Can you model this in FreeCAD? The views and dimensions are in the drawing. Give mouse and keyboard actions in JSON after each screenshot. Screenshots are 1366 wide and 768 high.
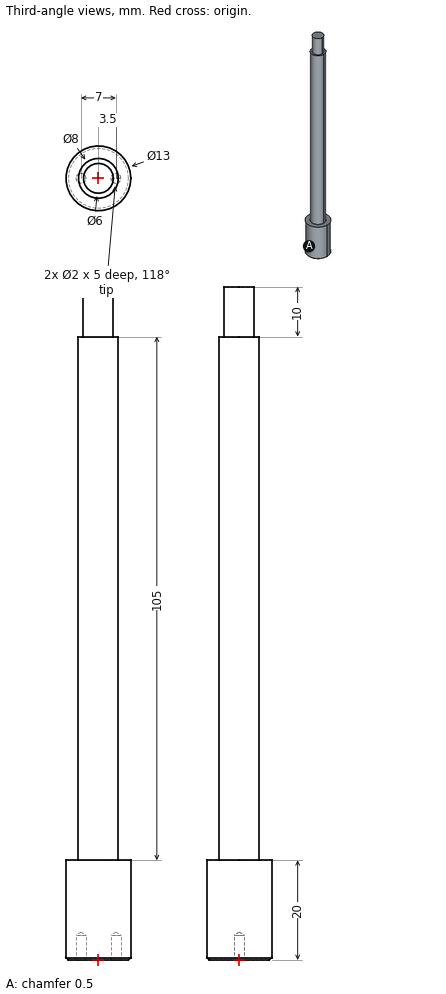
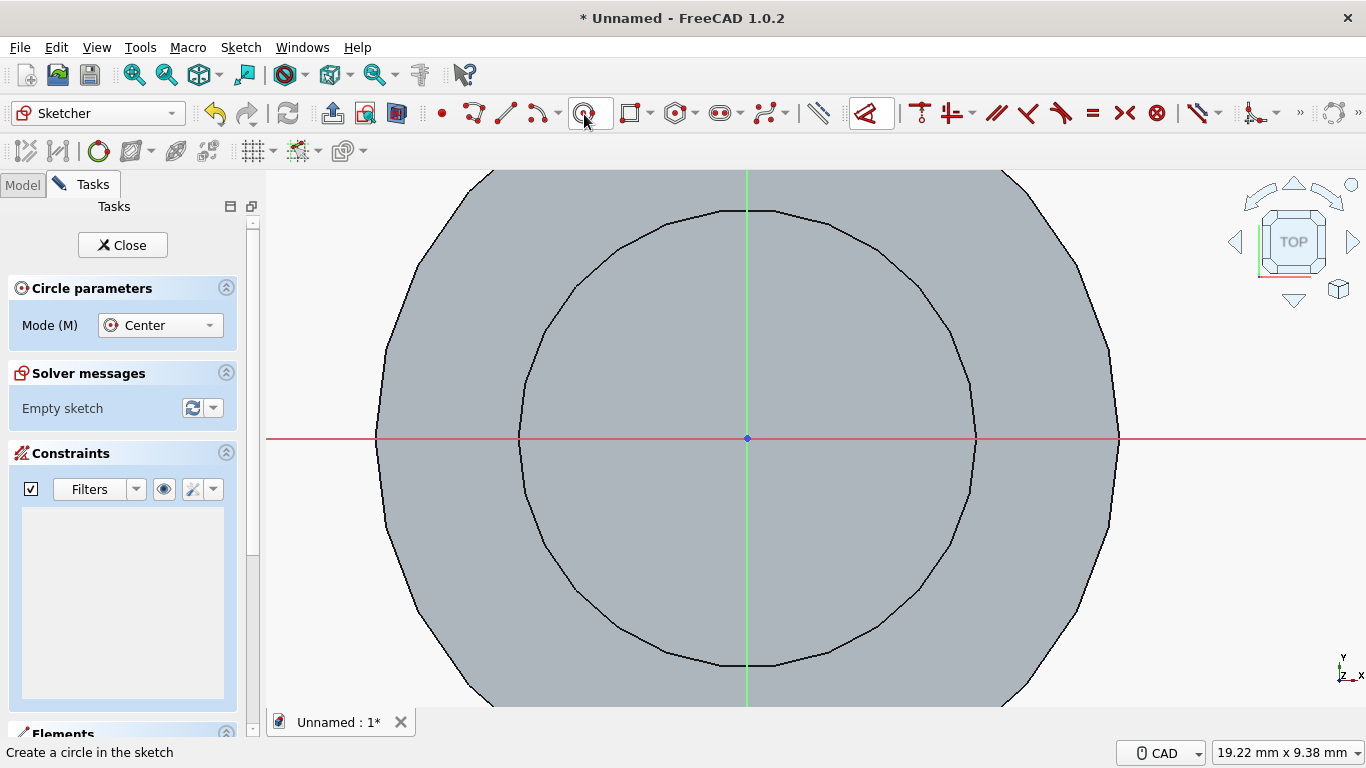
{"action": "left_click", "coordinate": [747, 438]}
{"action": "left_click", "coordinate": [869, 317]}
{"action": "key", "text": "Escape"}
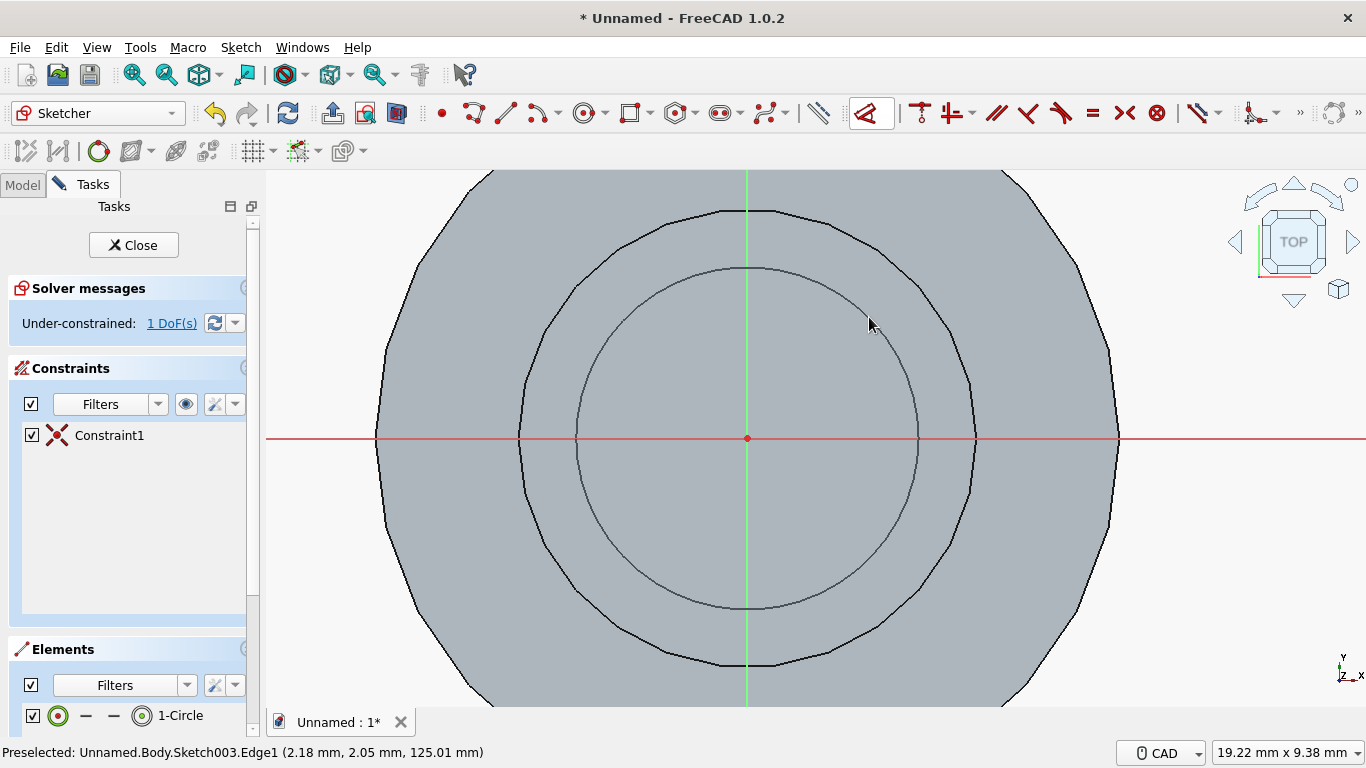
{"action": "left_click", "coordinate": [868, 317]}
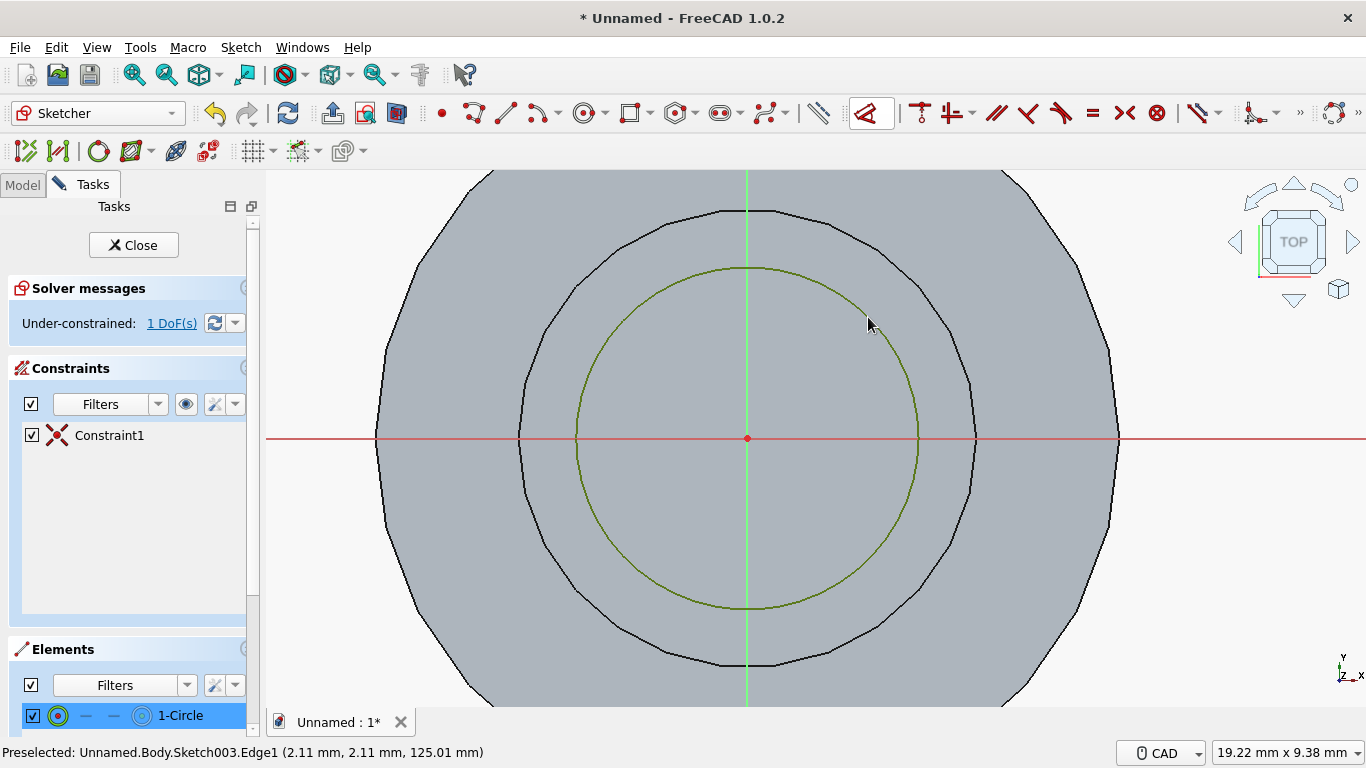
{"action": "key", "text": "k o"}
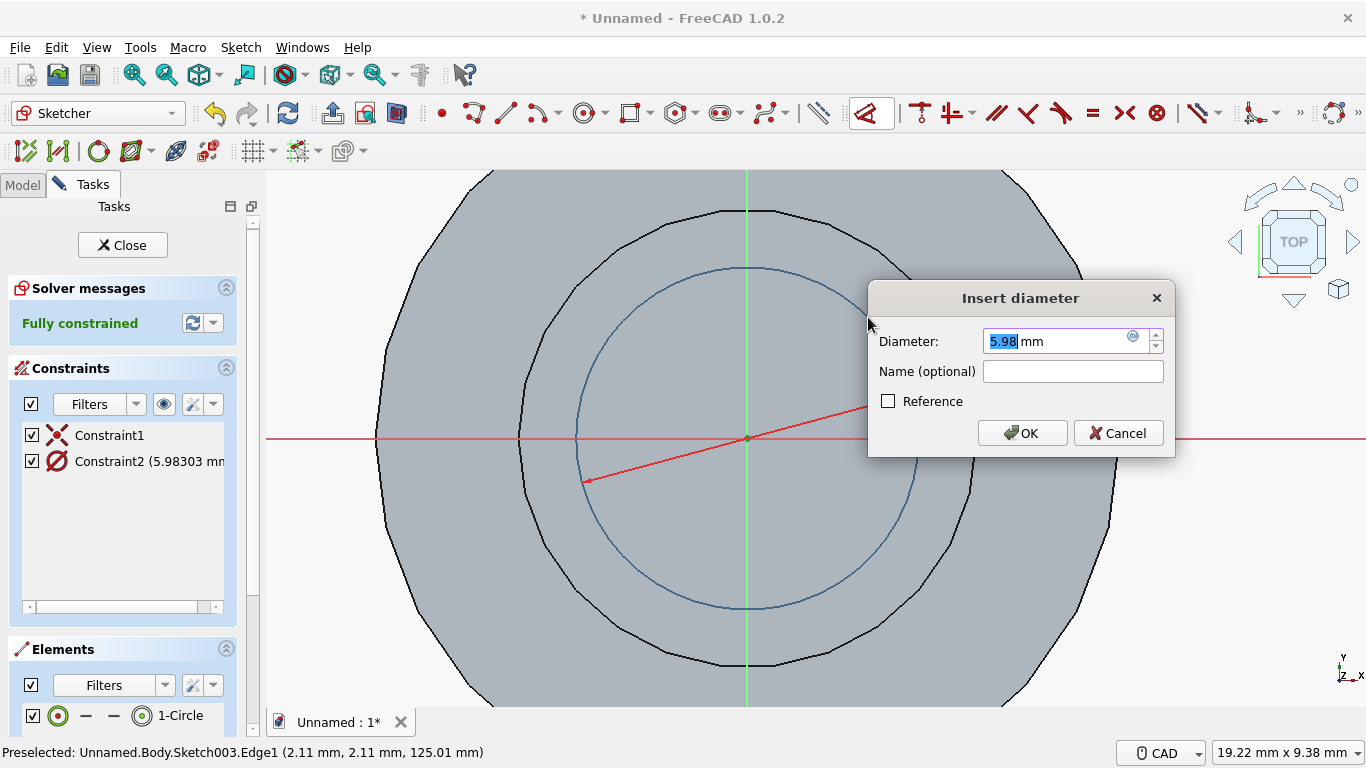
{"action": "type", "text": "6"}
{"action": "key", "text": "Return"}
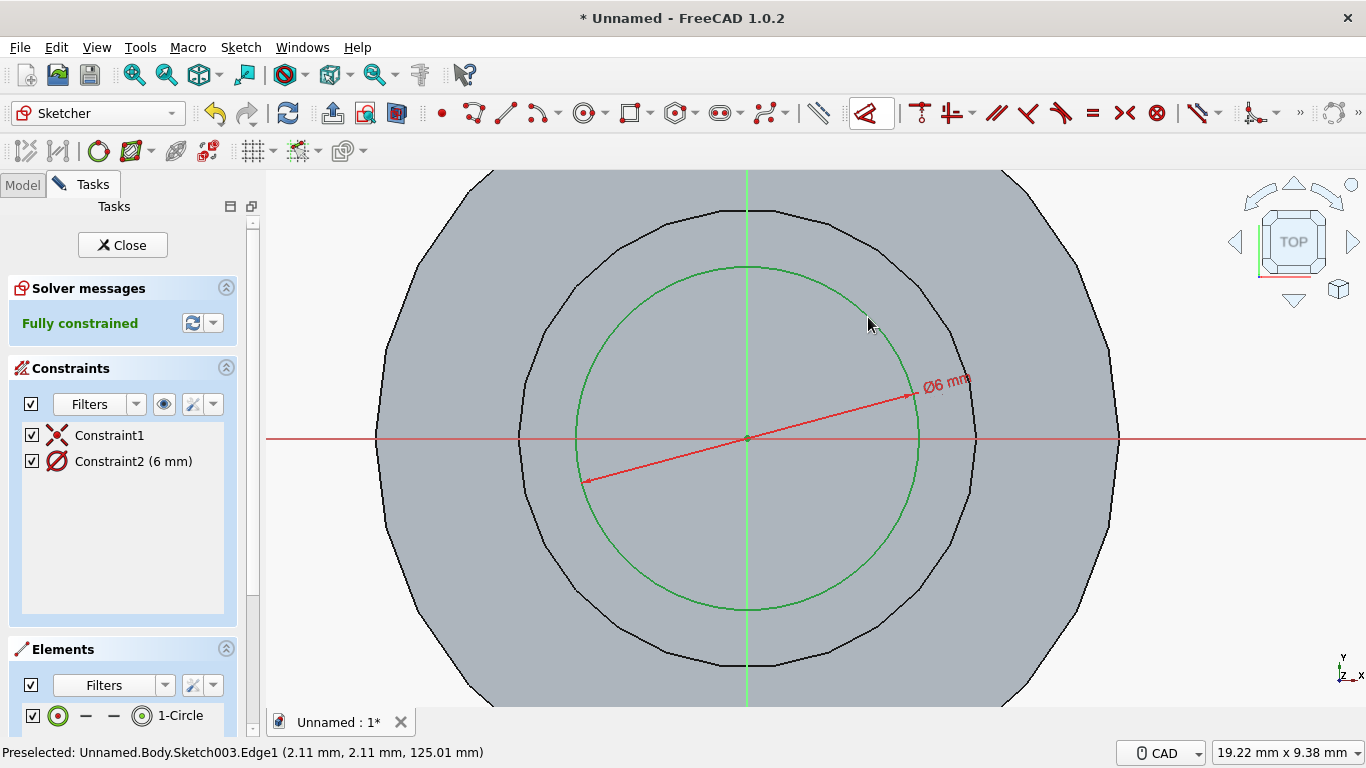
{"action": "left_click", "coordinate": [123, 245]}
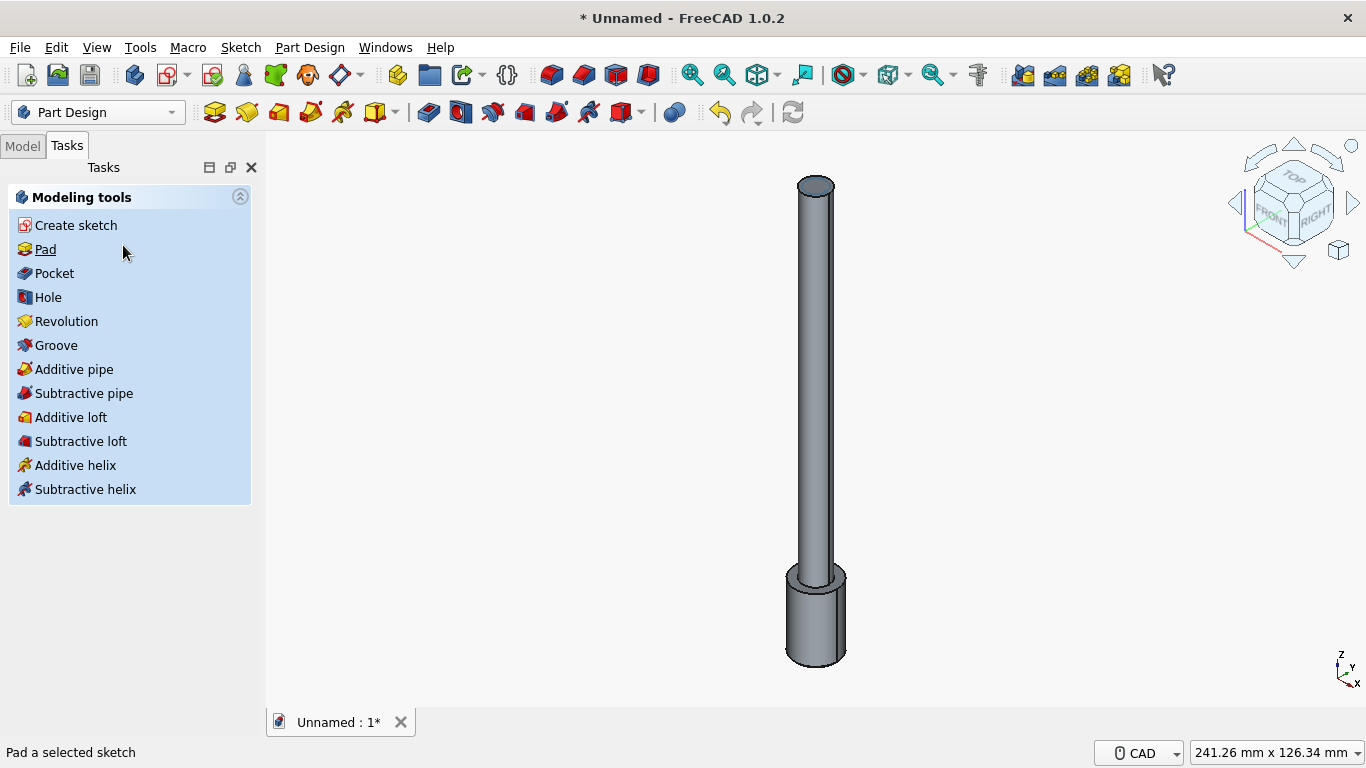
{"action": "left_click", "coordinate": [216, 112]}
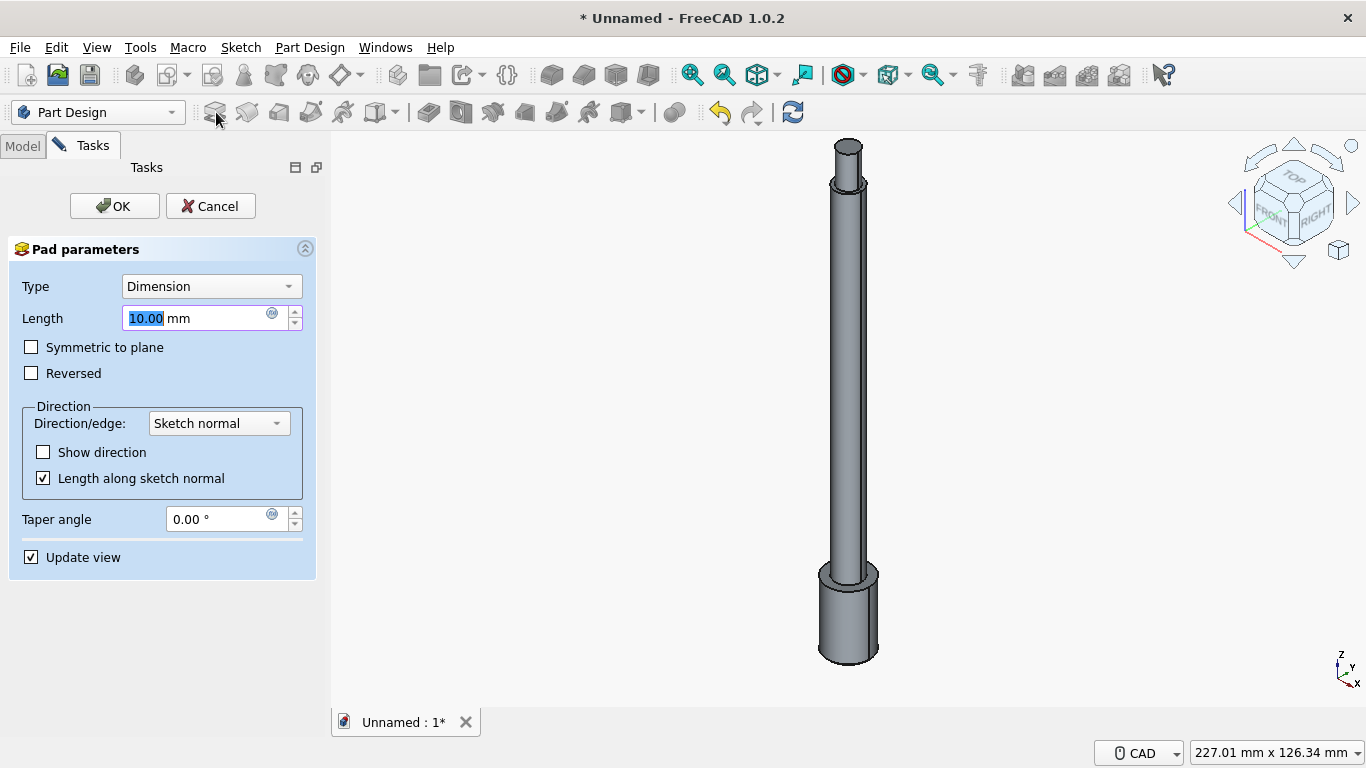
{"action": "type", "text": "10"}
{"action": "key", "text": "Tab"}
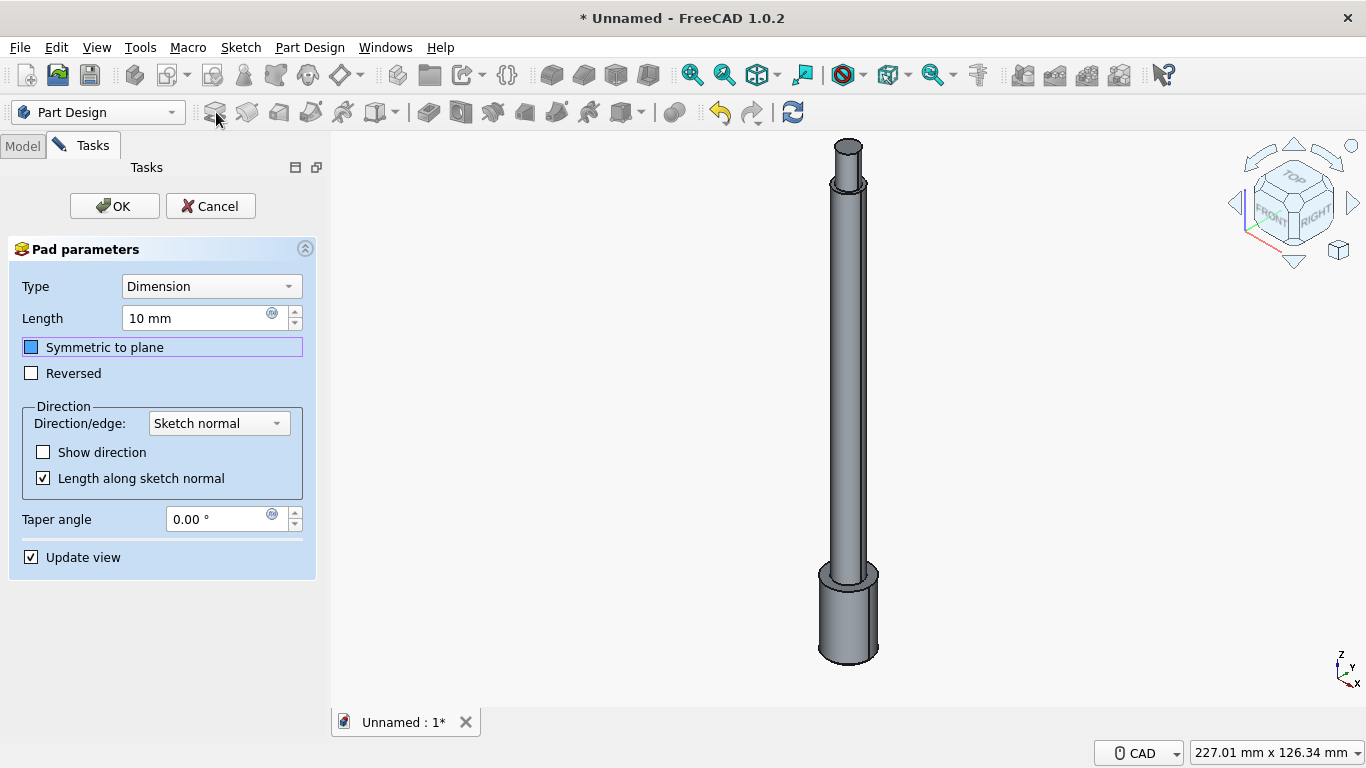
{"action": "left_click", "coordinate": [115, 206]}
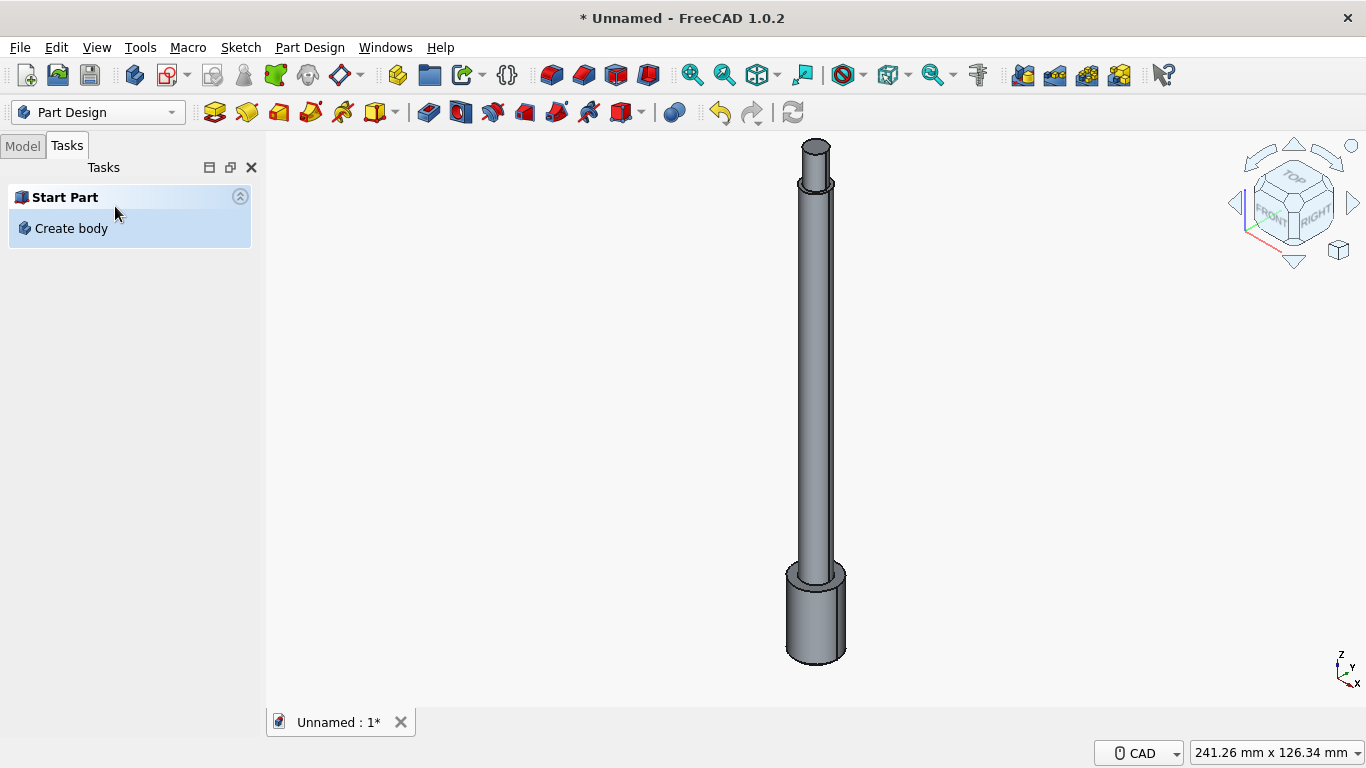
{"action": "key", "text": "v f"}